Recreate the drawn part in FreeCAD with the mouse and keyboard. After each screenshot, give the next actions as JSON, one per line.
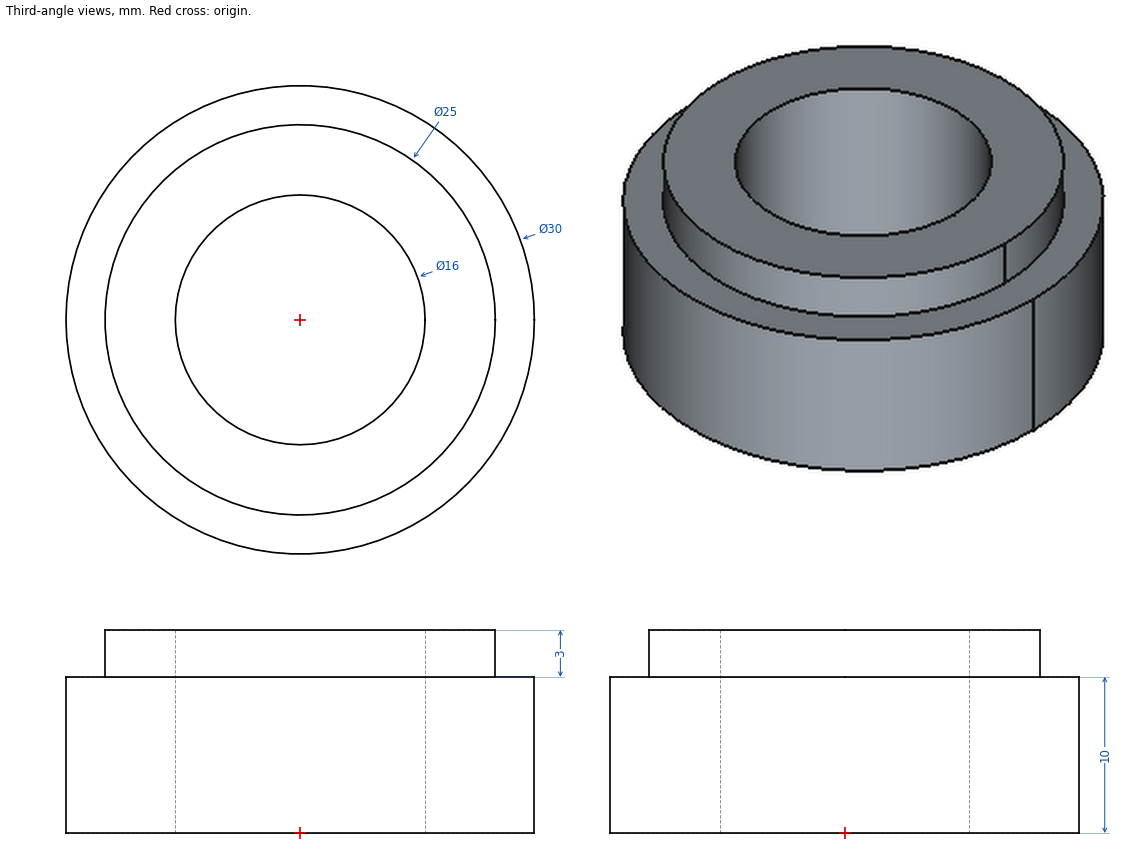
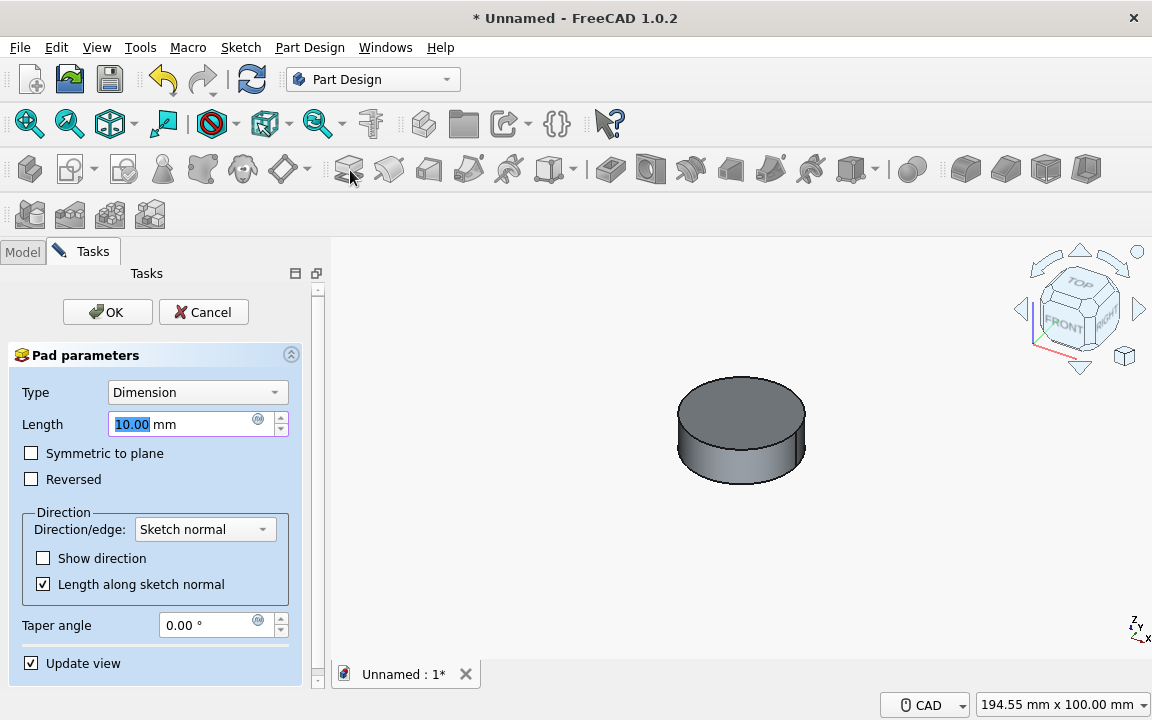
{"action": "type", "text": "10"}
{"action": "key", "text": "Tab"}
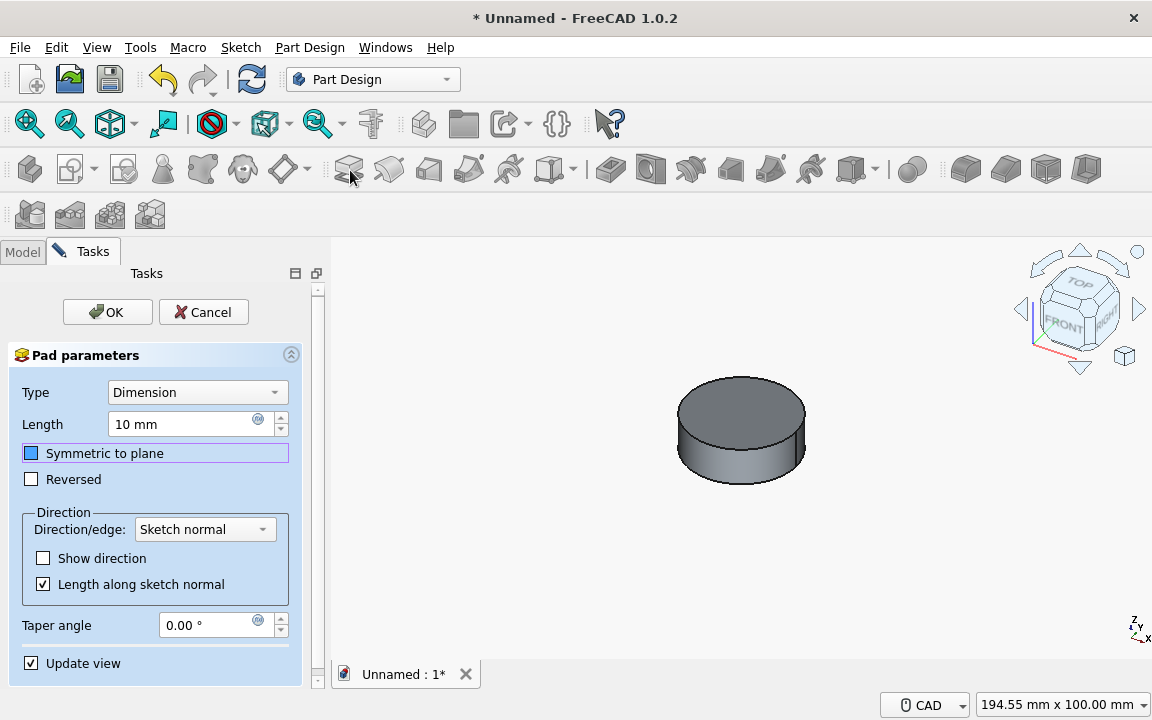
{"action": "left_click", "coordinate": [108, 312]}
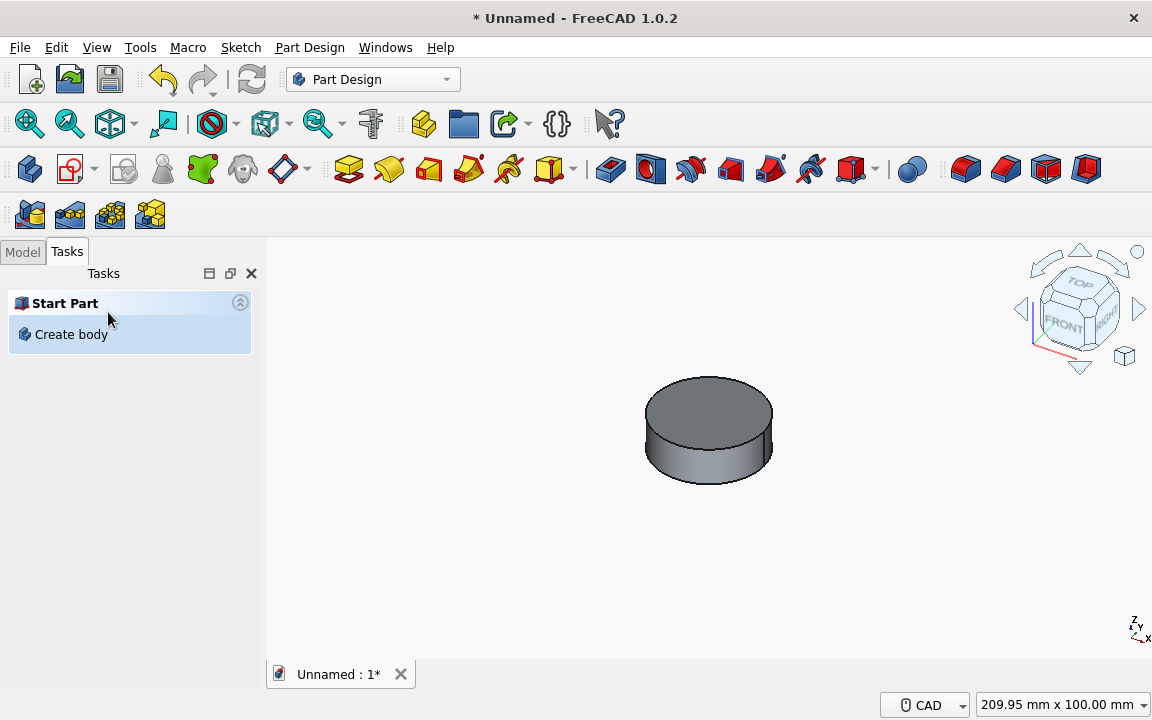
{"action": "left_click", "coordinate": [30, 124]}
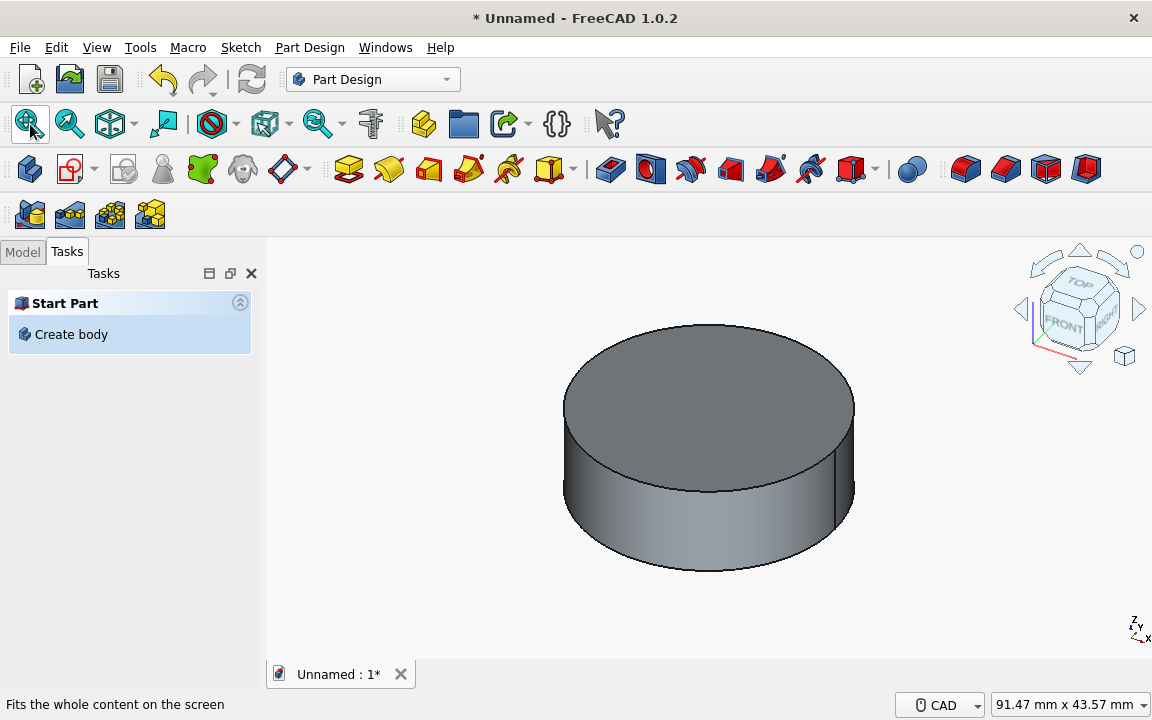
{"action": "left_click", "coordinate": [709, 407]}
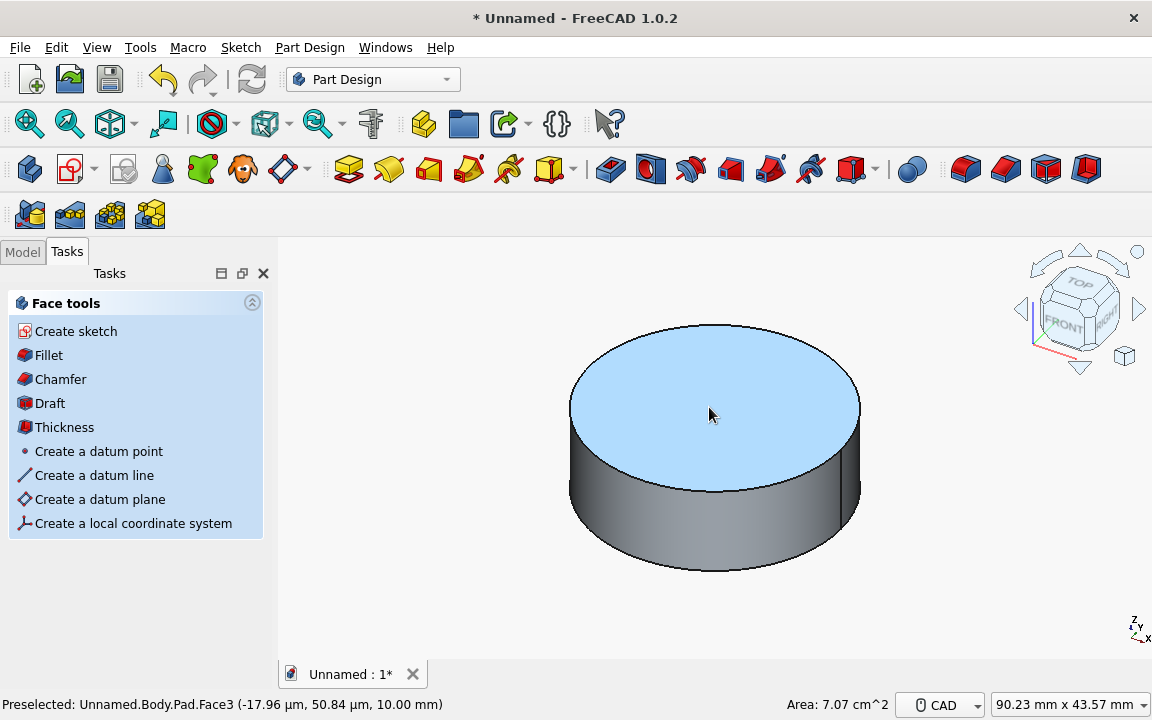
{"action": "left_click", "coordinate": [70, 170]}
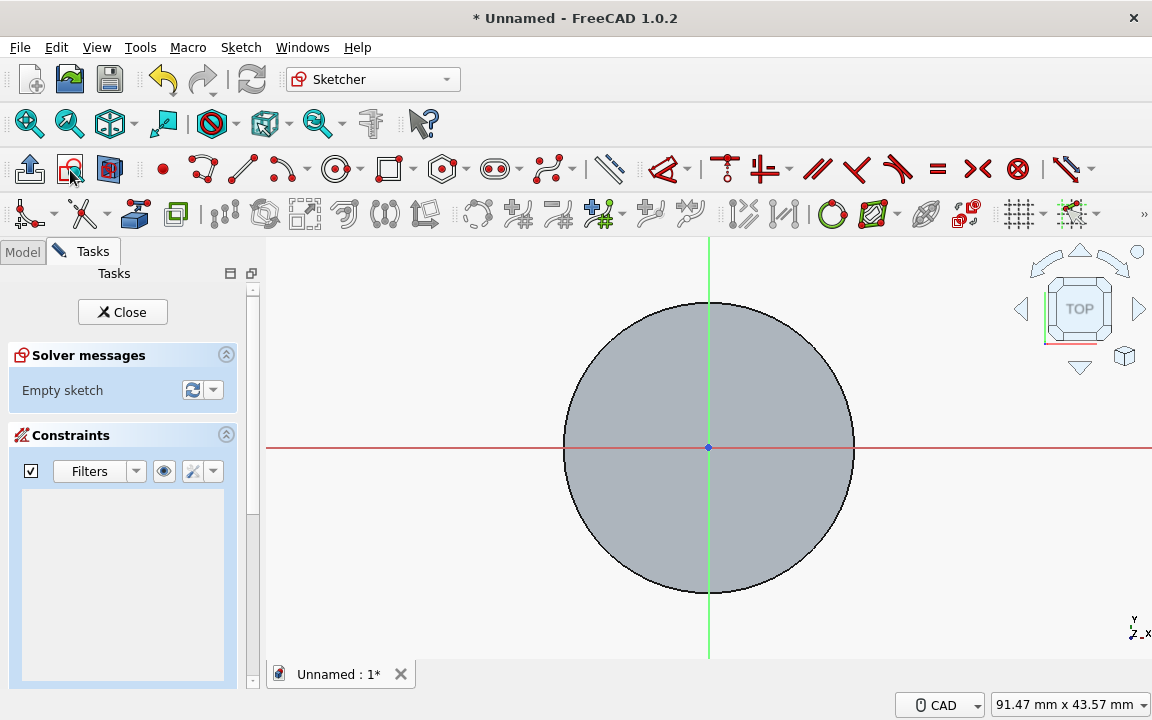
{"action": "key", "text": "g c"}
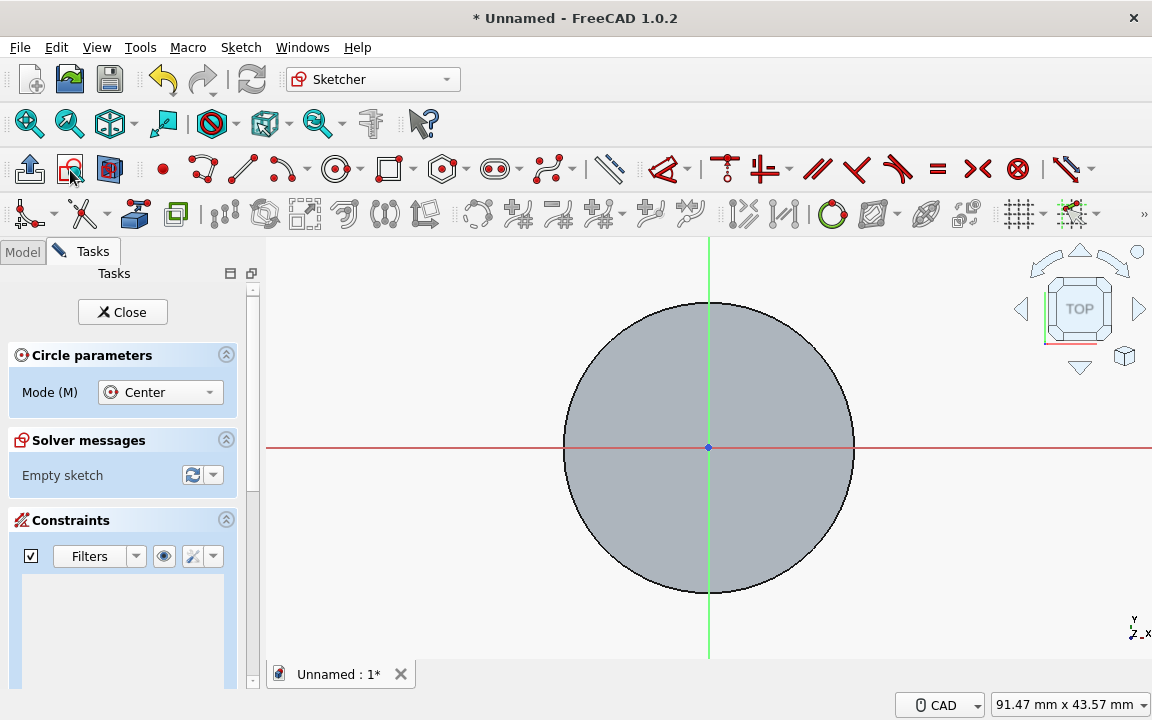
{"action": "left_click", "coordinate": [709, 448]}
{"action": "left_click", "coordinate": [795, 362]}
{"action": "key", "text": "Escape"}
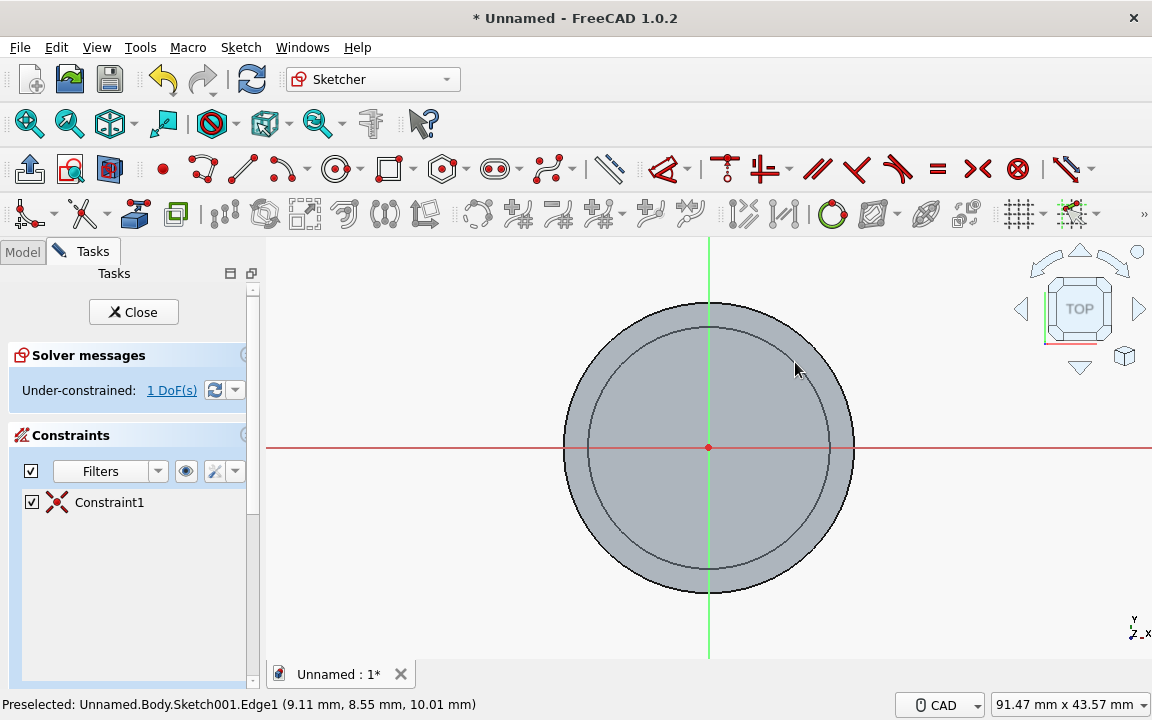
{"action": "left_click", "coordinate": [794, 362]}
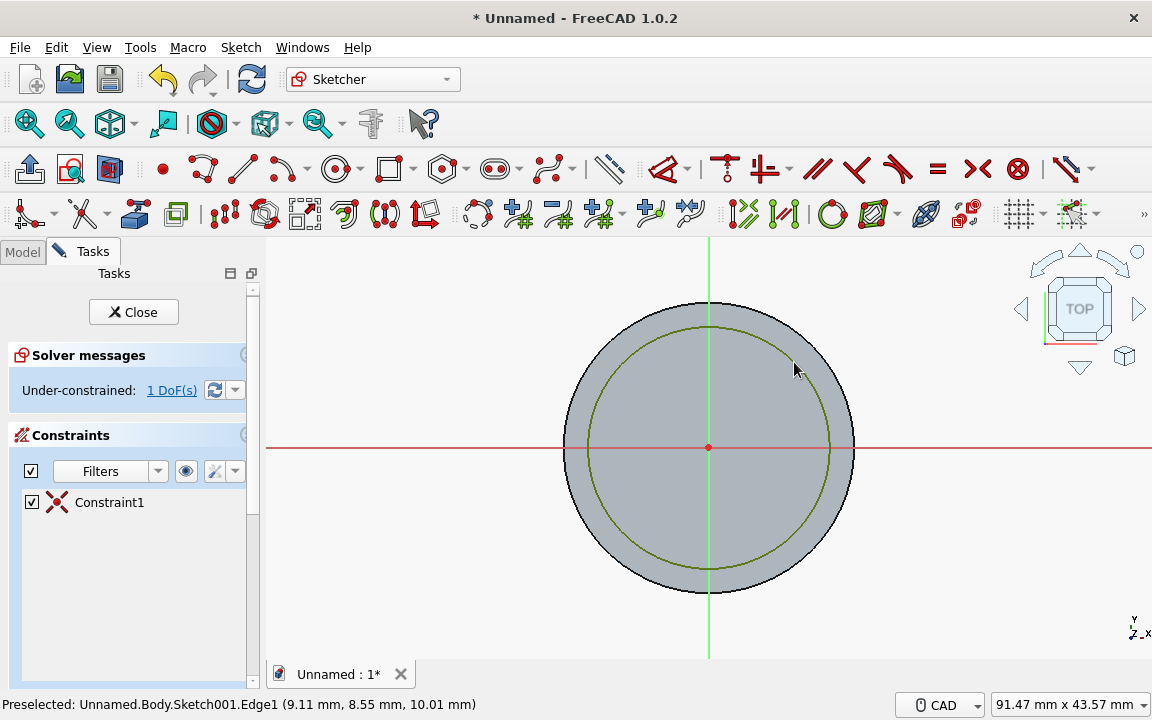
{"action": "key", "text": "k o"}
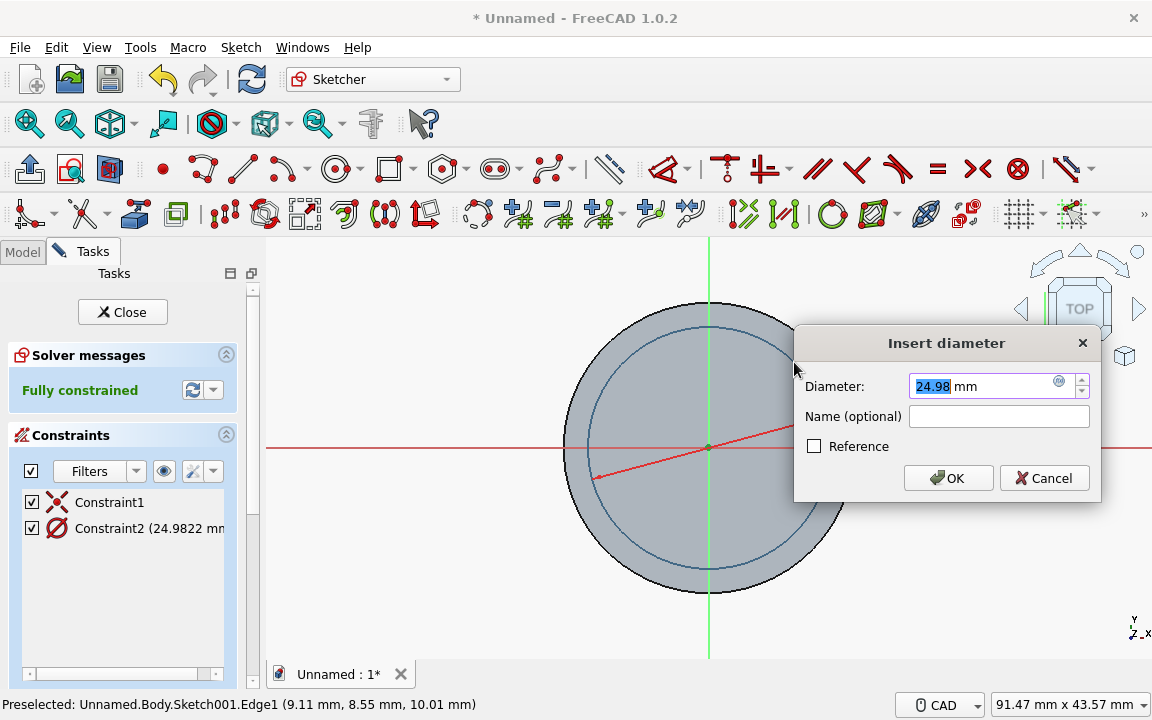
{"action": "type", "text": "25"}
{"action": "key", "text": "Return"}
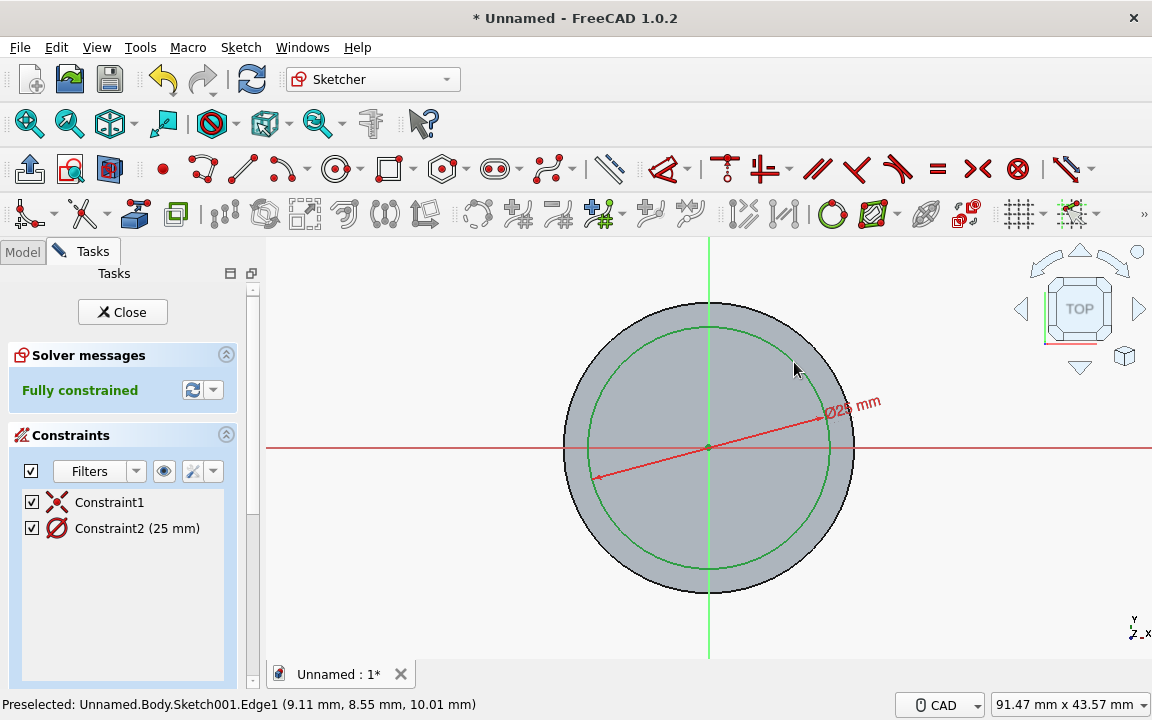
{"action": "left_click", "coordinate": [123, 312]}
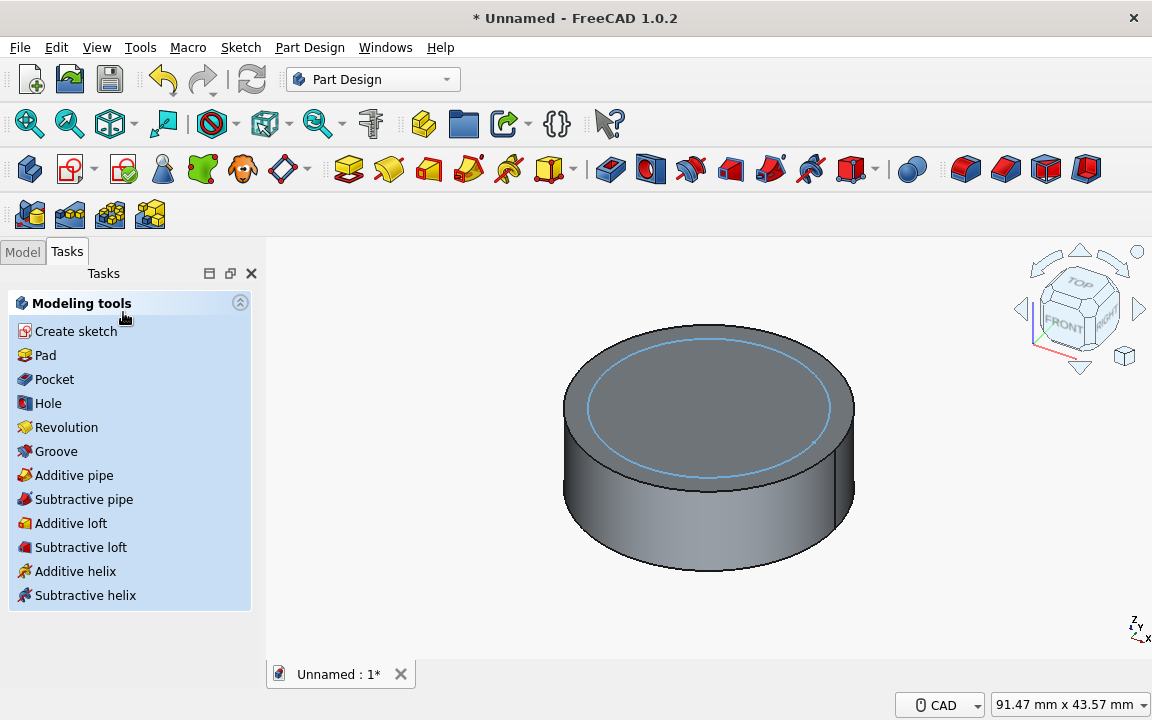
{"action": "left_click", "coordinate": [350, 170]}